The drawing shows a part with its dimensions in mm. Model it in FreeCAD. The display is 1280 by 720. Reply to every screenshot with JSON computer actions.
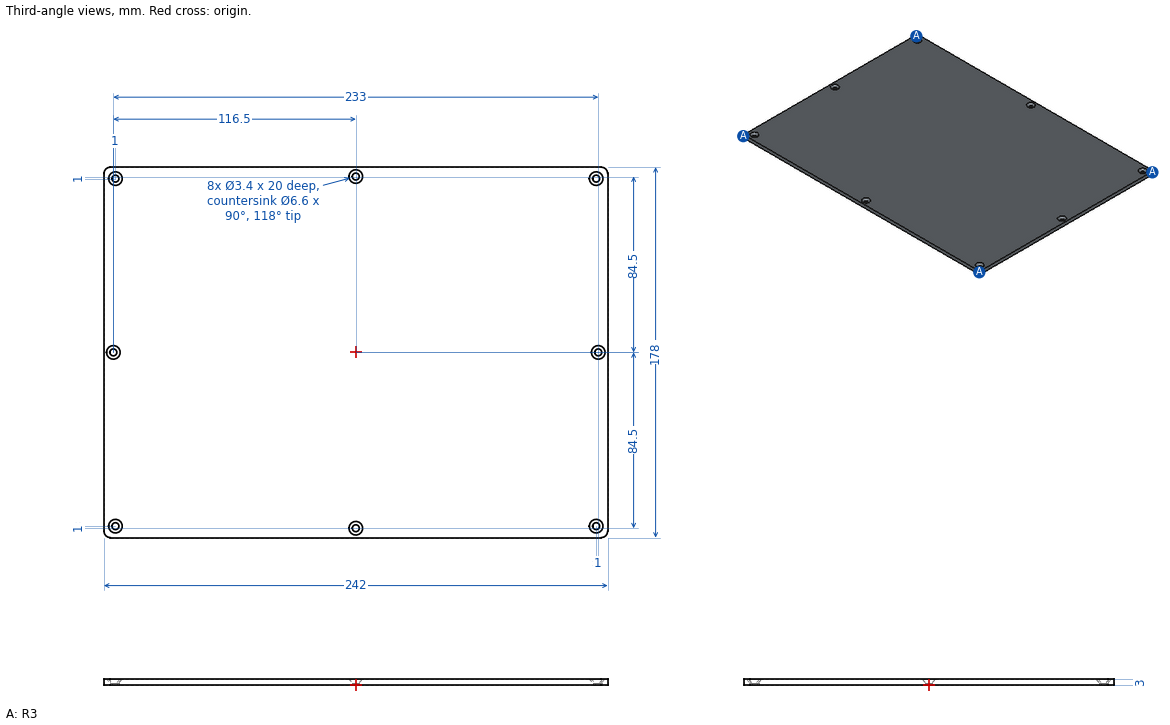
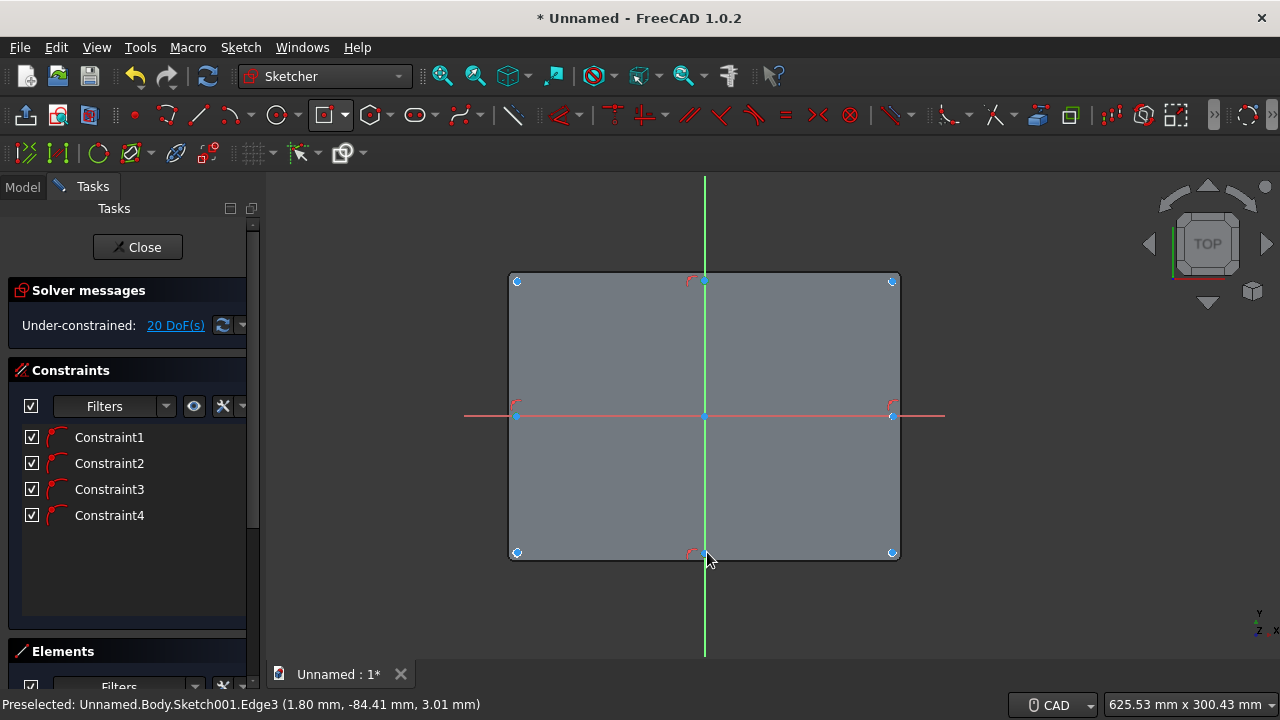
{"action": "scroll", "coordinate": [895, 414], "scroll_direction": "up", "scroll_amount": 10}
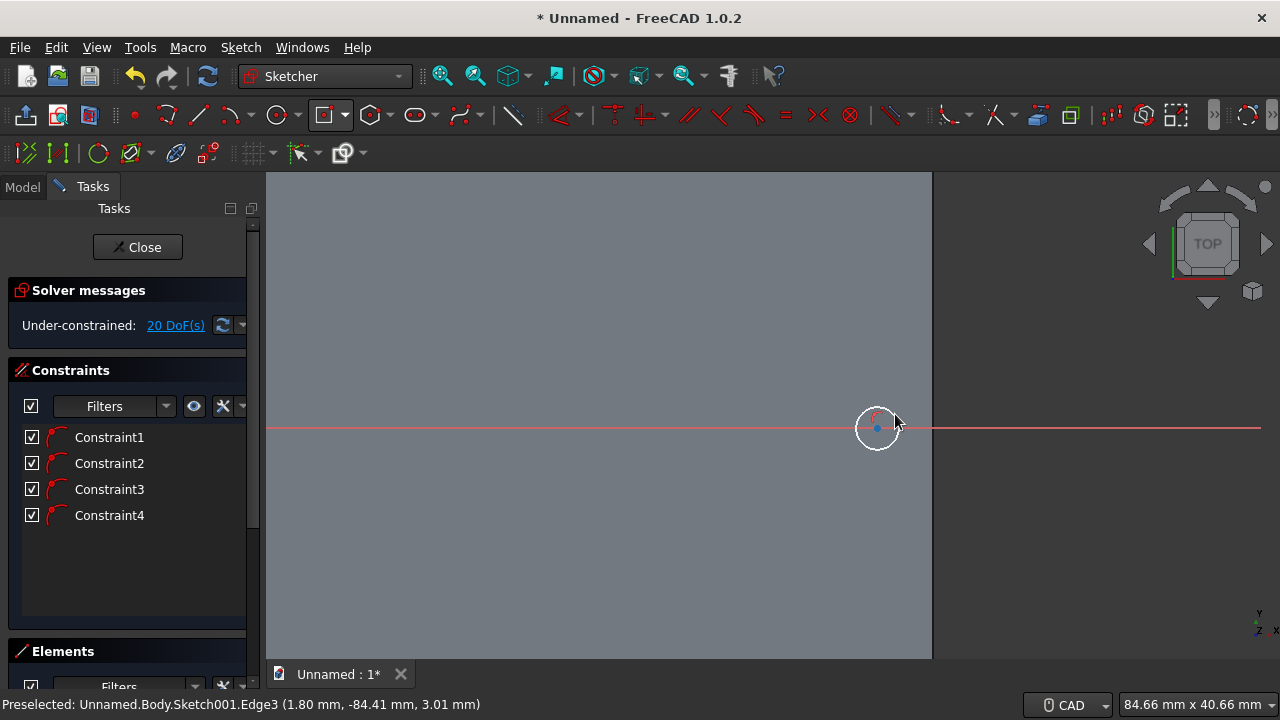
{"action": "left_click", "coordinate": [892, 413]}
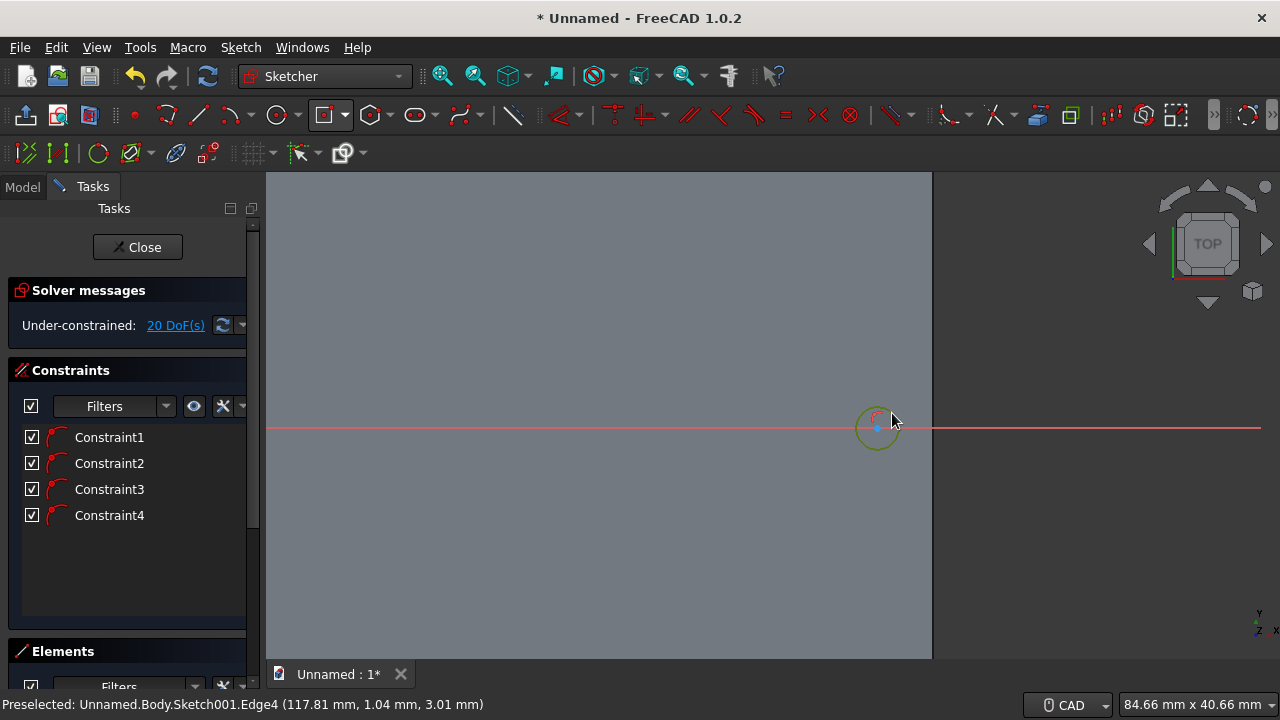
{"action": "scroll", "coordinate": [896, 413], "scroll_direction": "down", "scroll_amount": 10}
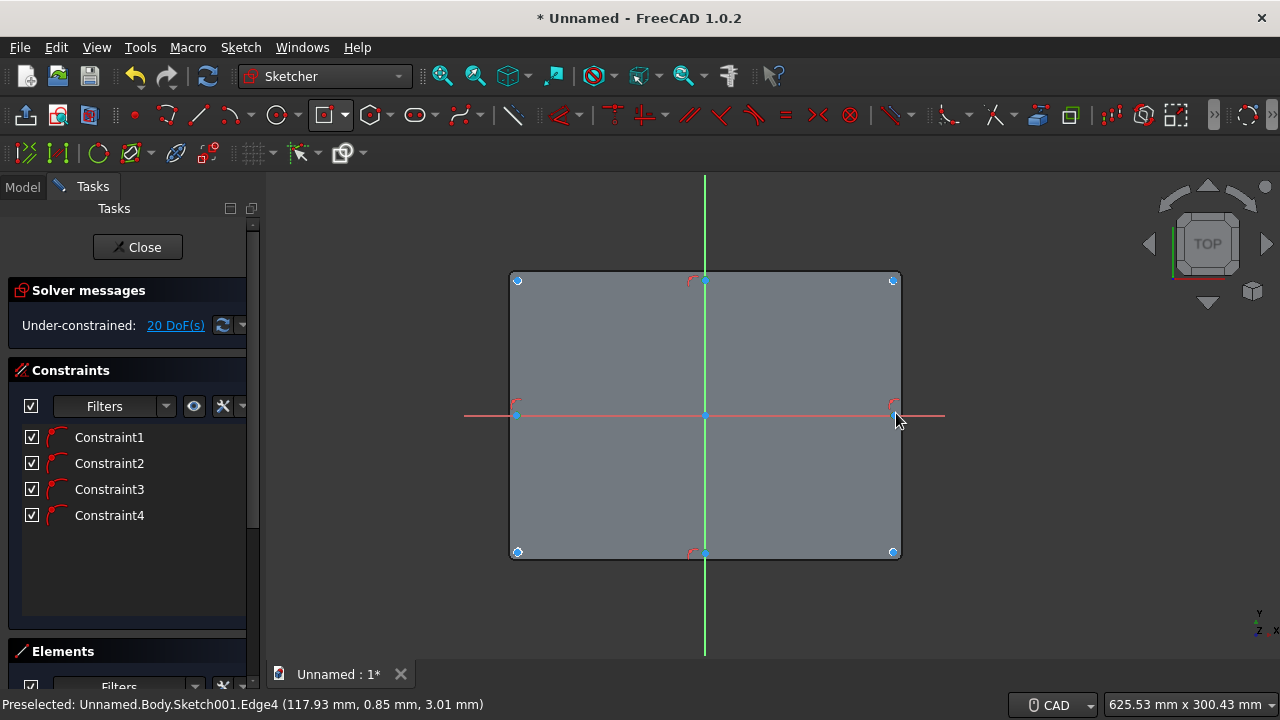
{"action": "scroll", "coordinate": [520, 279], "scroll_direction": "up", "scroll_amount": 7}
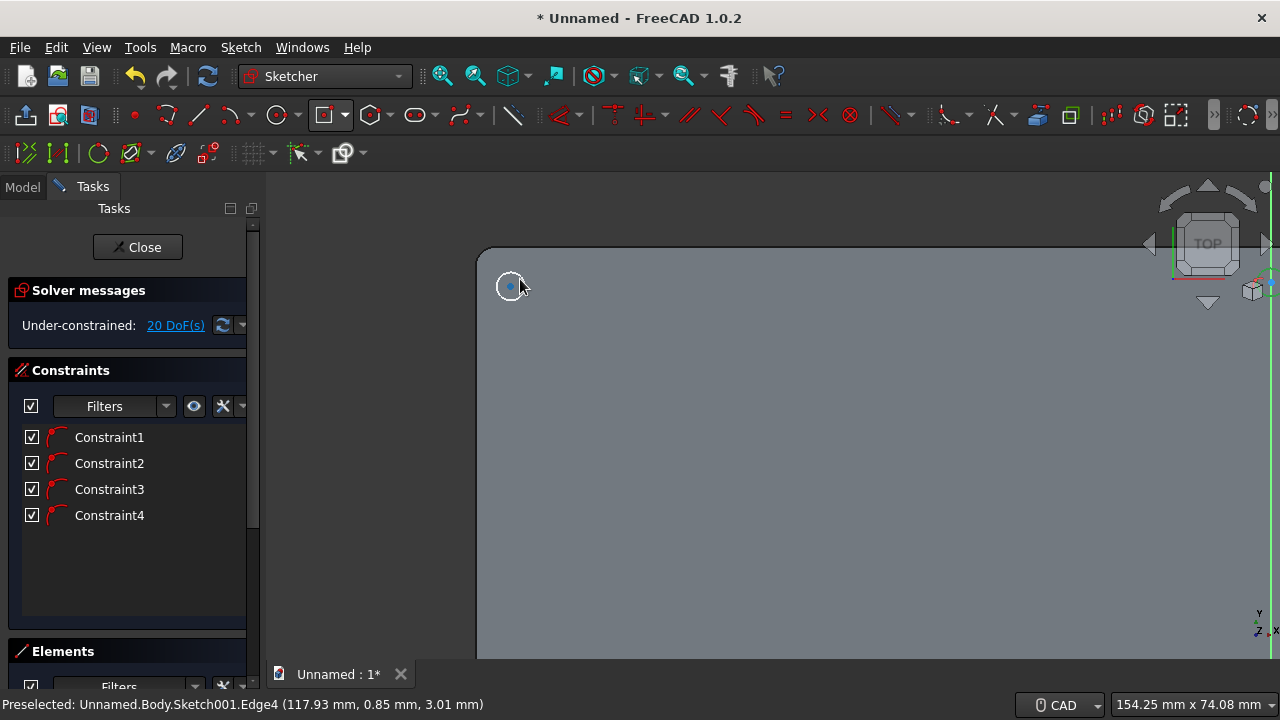
{"action": "left_click", "coordinate": [521, 277]}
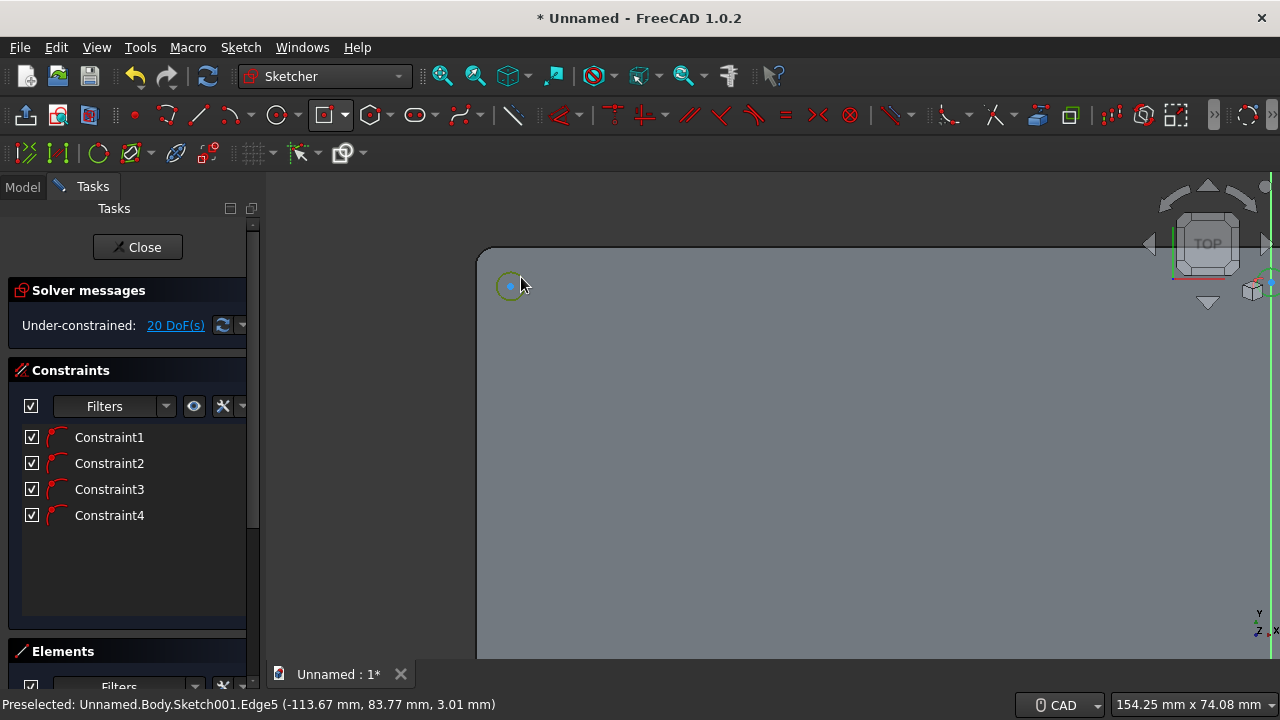
{"action": "scroll", "coordinate": [519, 279], "scroll_direction": "down", "scroll_amount": 7}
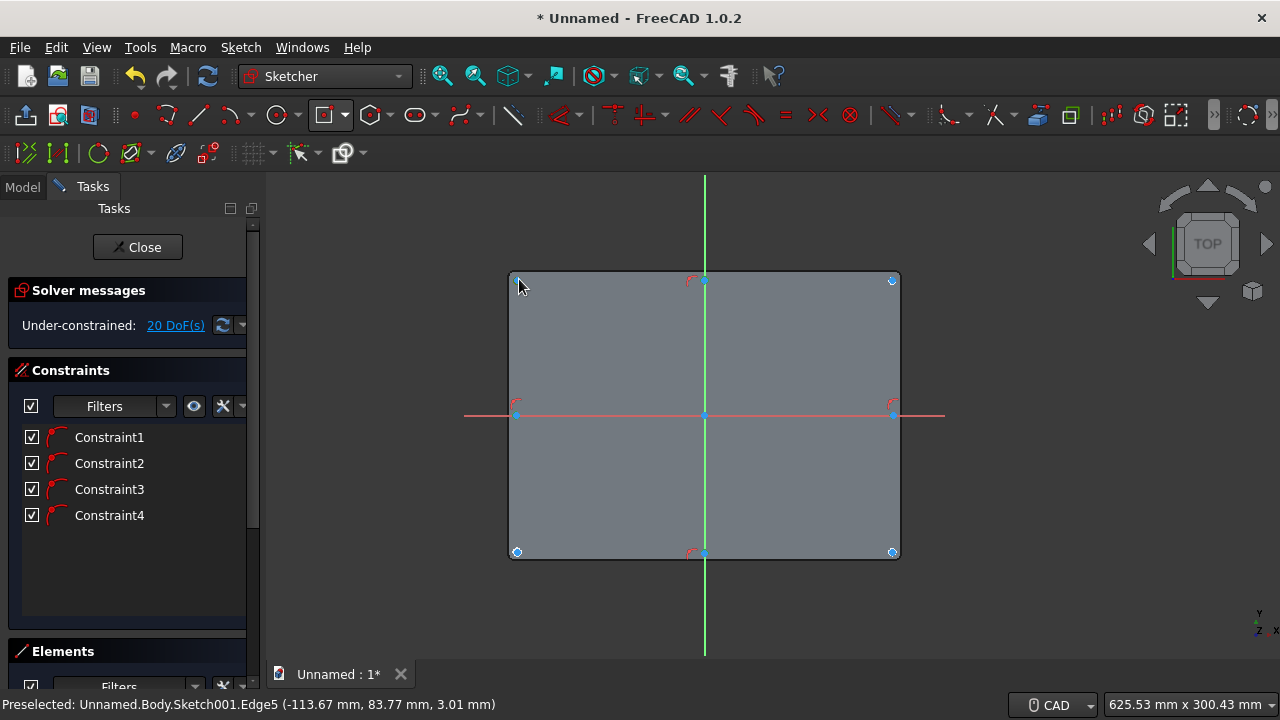
{"action": "scroll", "coordinate": [520, 549], "scroll_direction": "up", "scroll_amount": 7}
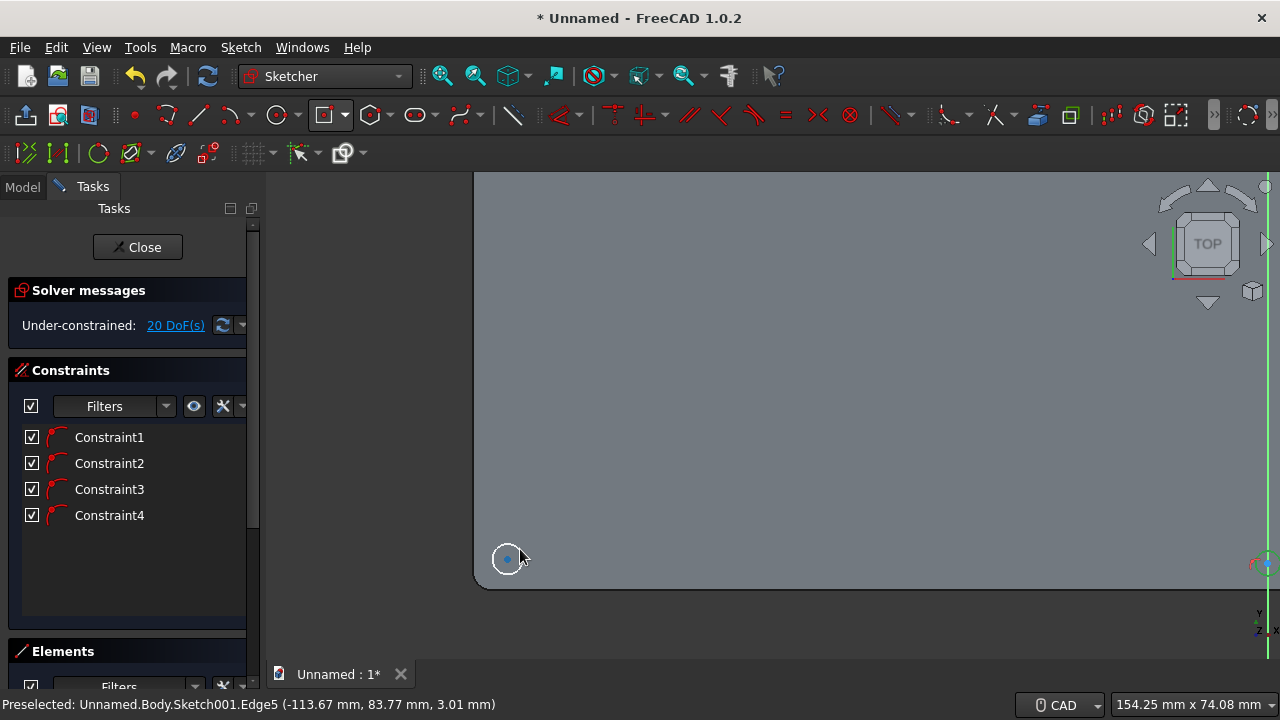
{"action": "left_click", "coordinate": [518, 548]}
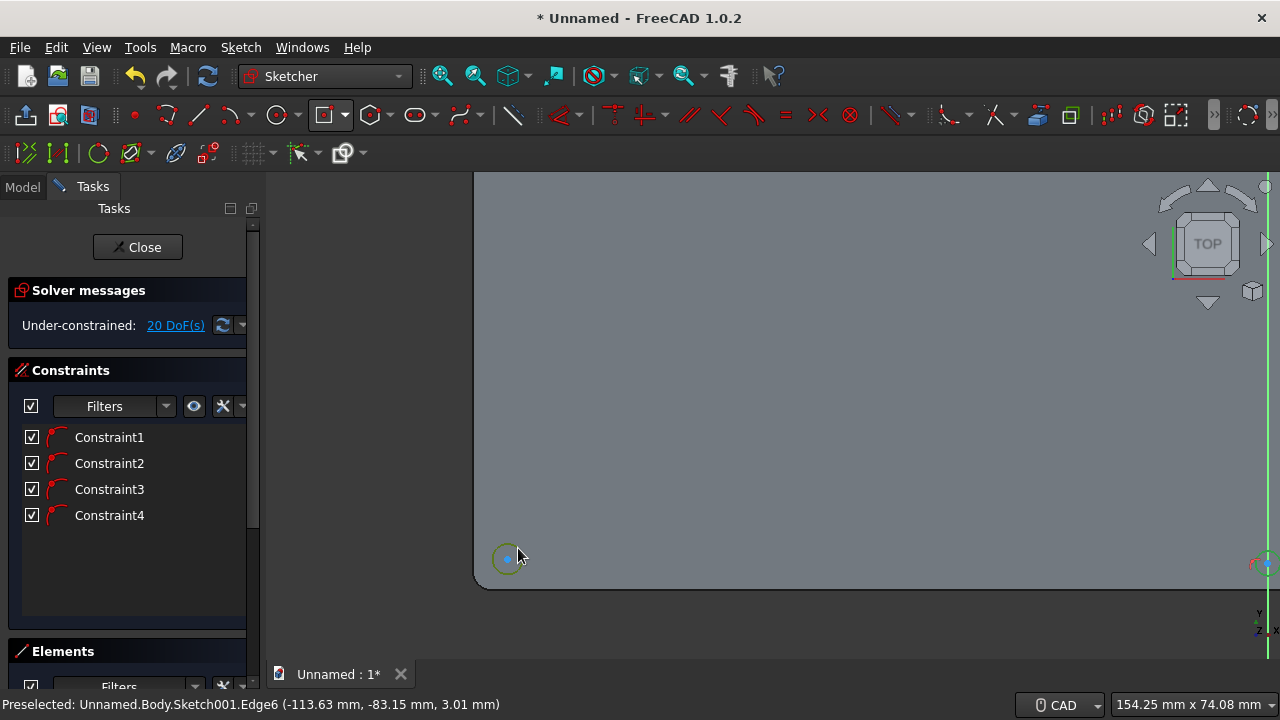
{"action": "scroll", "coordinate": [520, 550], "scroll_direction": "down", "scroll_amount": 7}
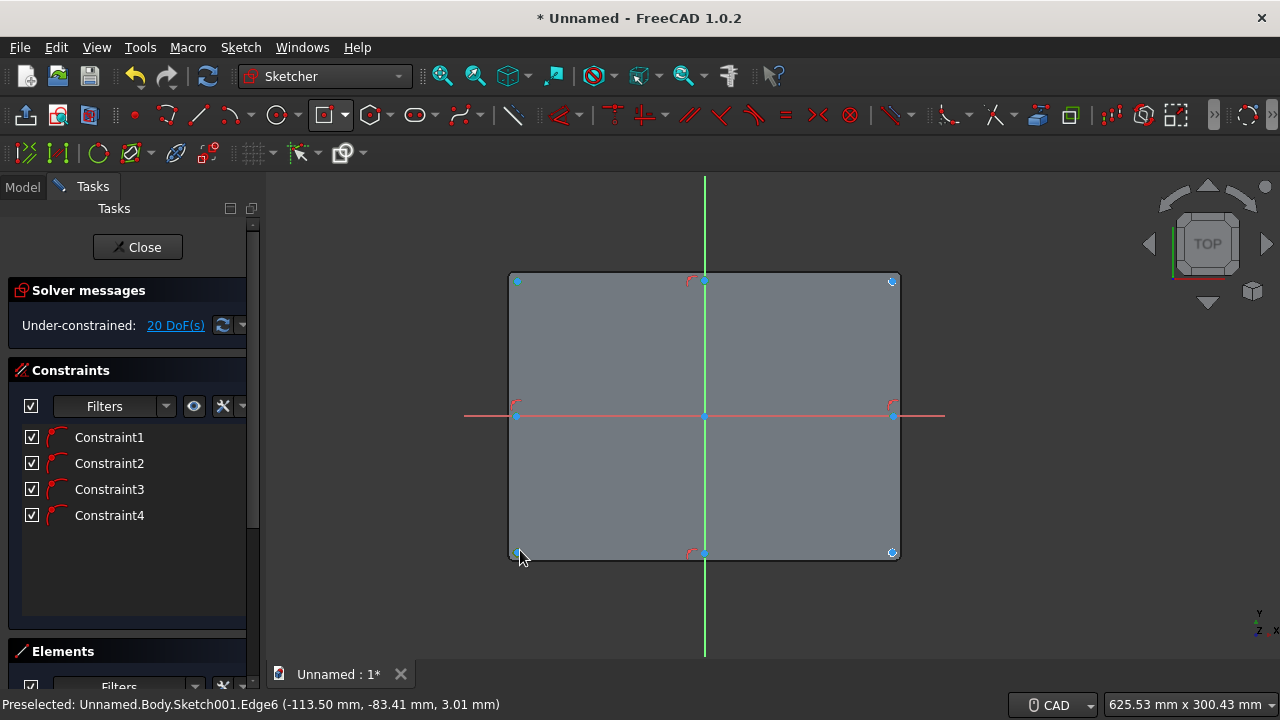
{"action": "scroll", "coordinate": [895, 550], "scroll_direction": "up", "scroll_amount": 8}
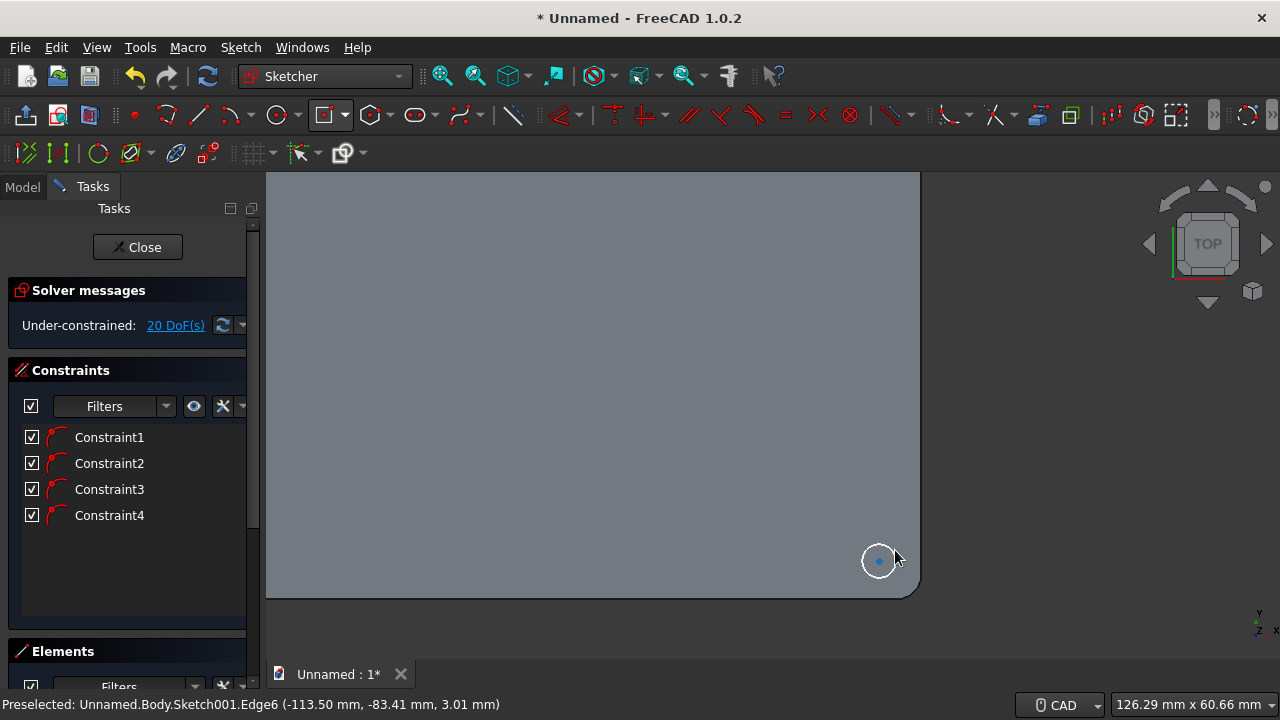
{"action": "left_click", "coordinate": [891, 549]}